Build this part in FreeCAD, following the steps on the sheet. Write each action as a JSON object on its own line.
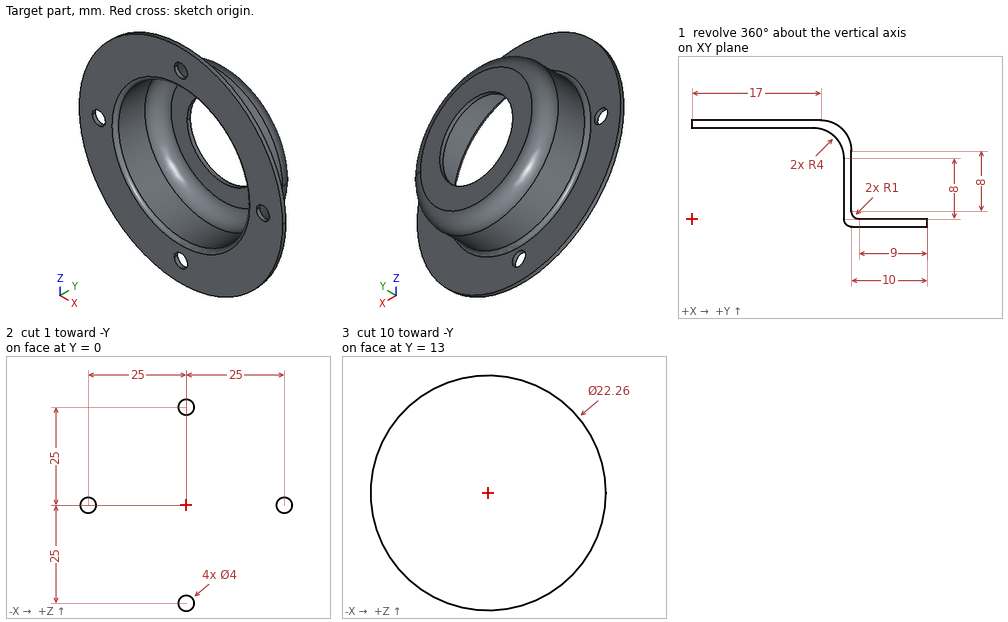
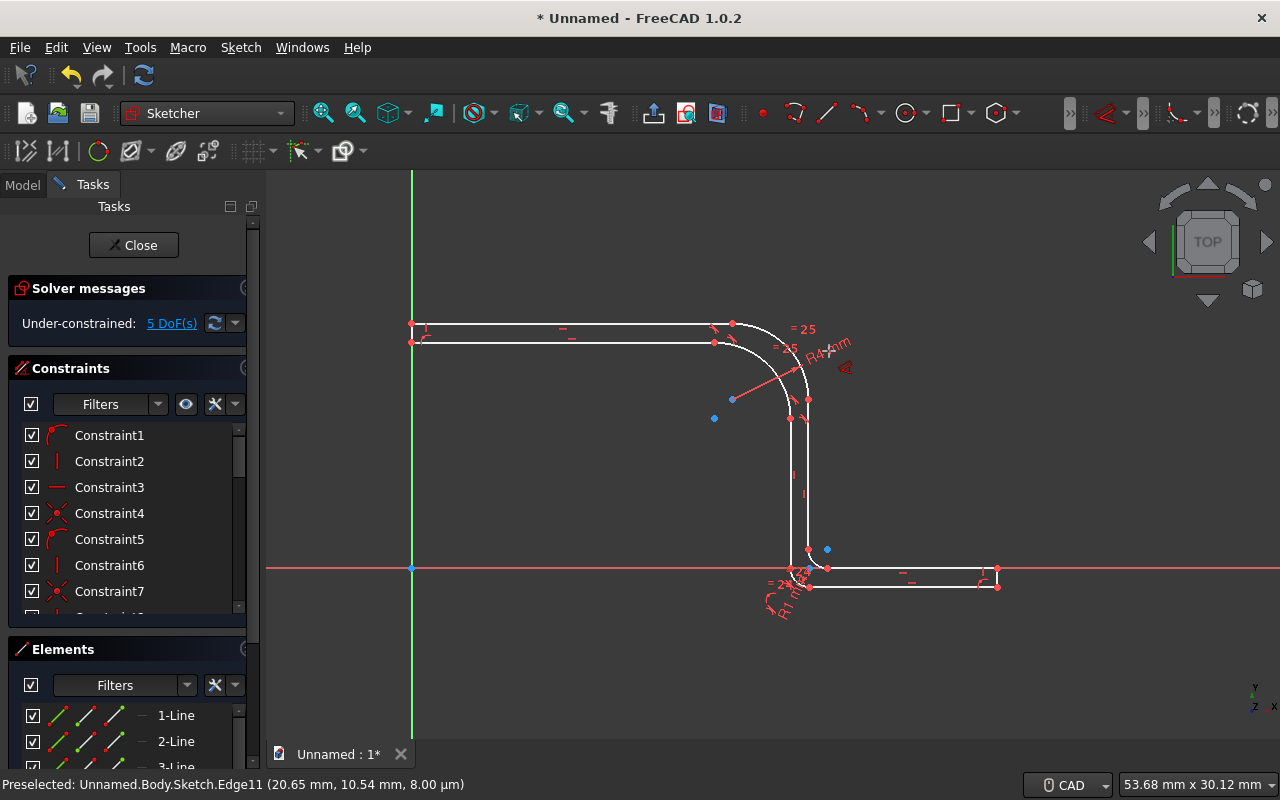
{"action": "left_click", "coordinate": [791, 463]}
{"action": "left_click", "coordinate": [825, 493]}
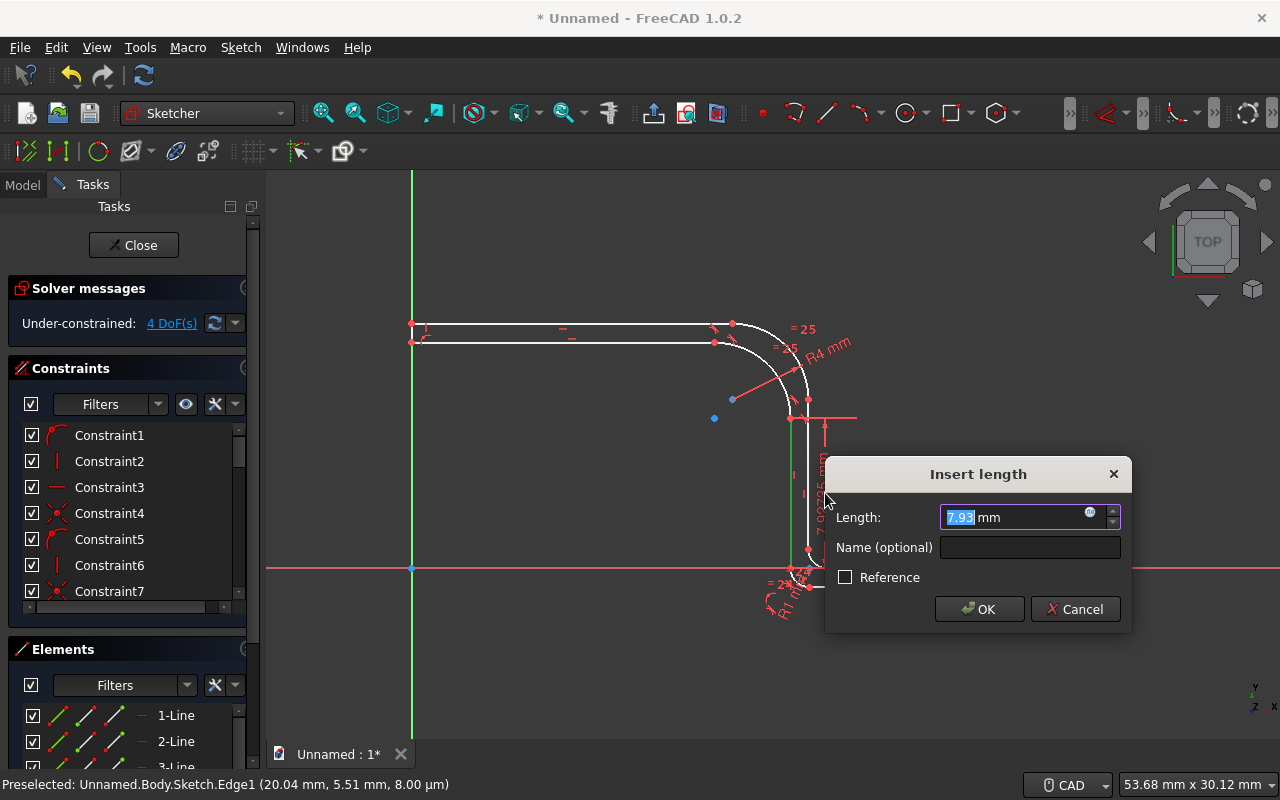
{"action": "type", "text": "8"}
{"action": "key", "text": "Return"}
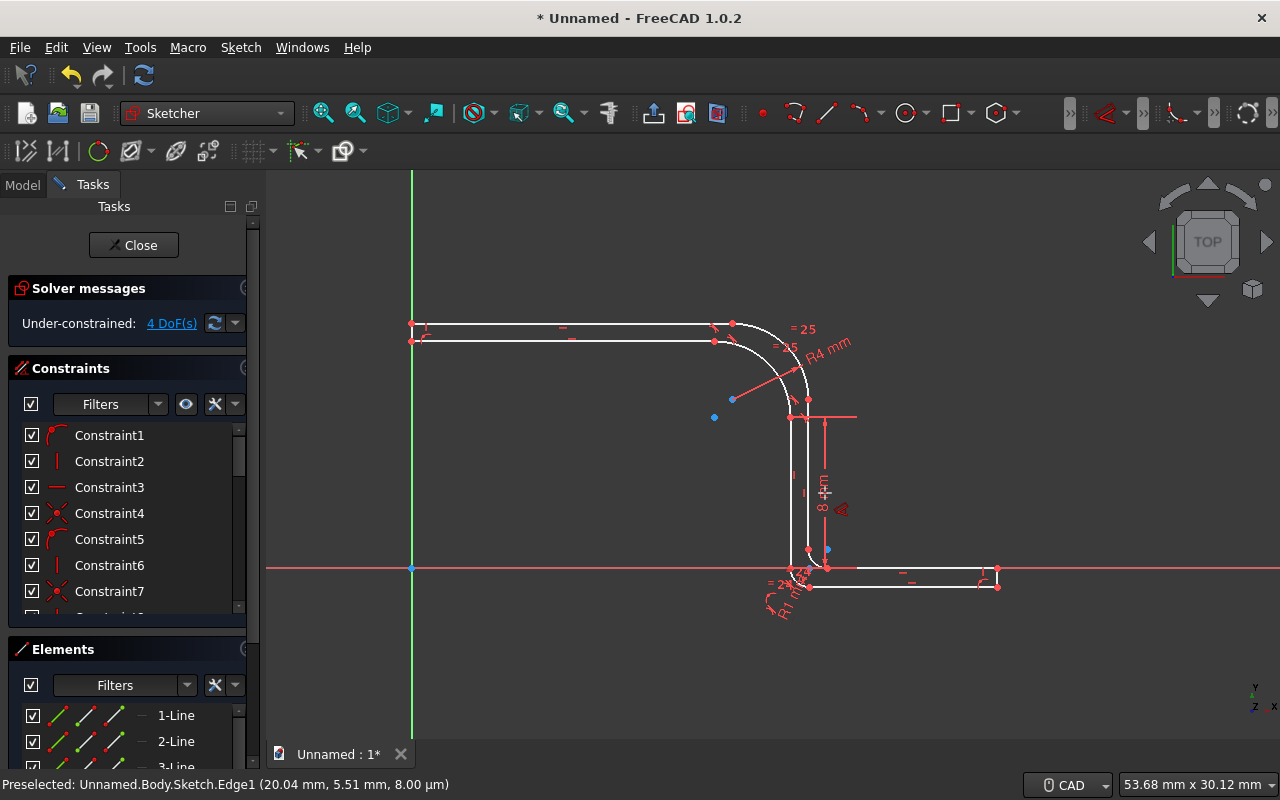
{"action": "left_click", "coordinate": [946, 568]}
{"action": "left_click", "coordinate": [912, 602]}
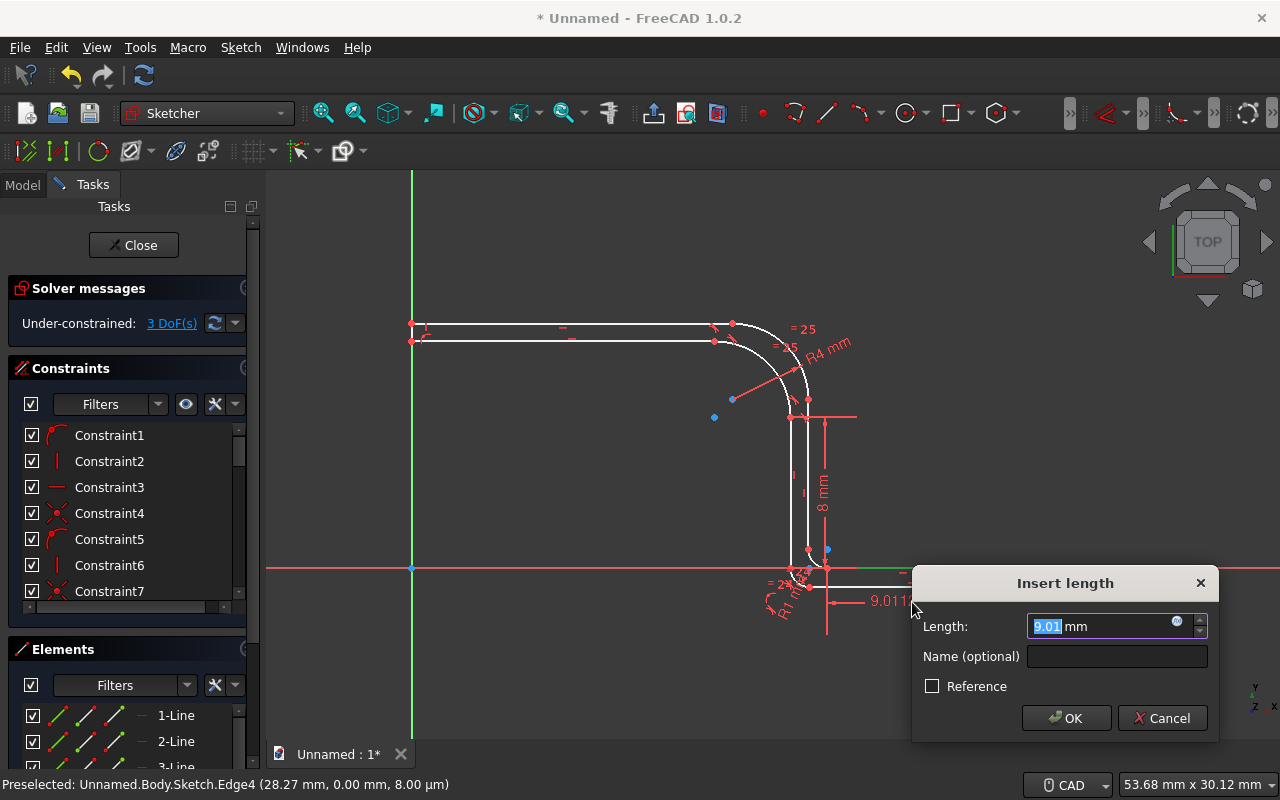
{"action": "type", "text": "9"}
{"action": "key", "text": "Return"}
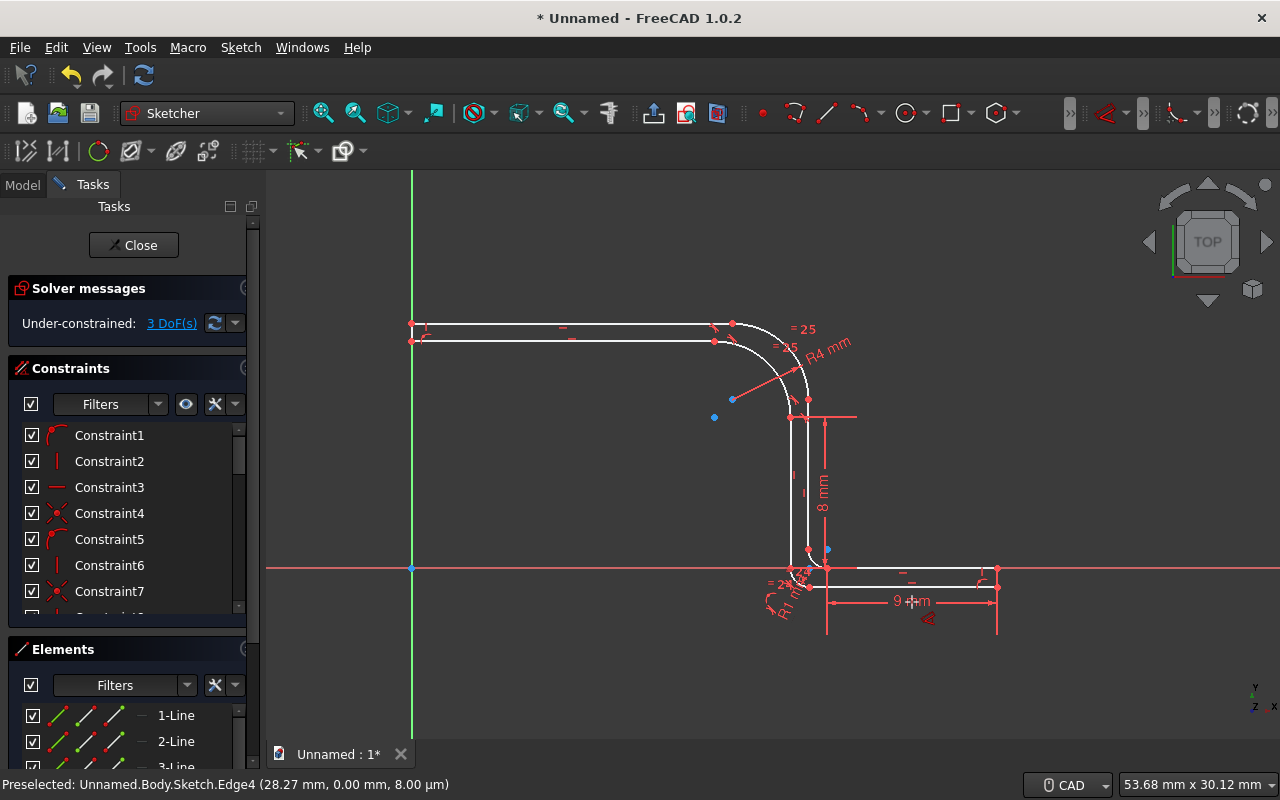
{"action": "left_click", "coordinate": [808, 504]}
{"action": "left_click", "coordinate": [842, 440]}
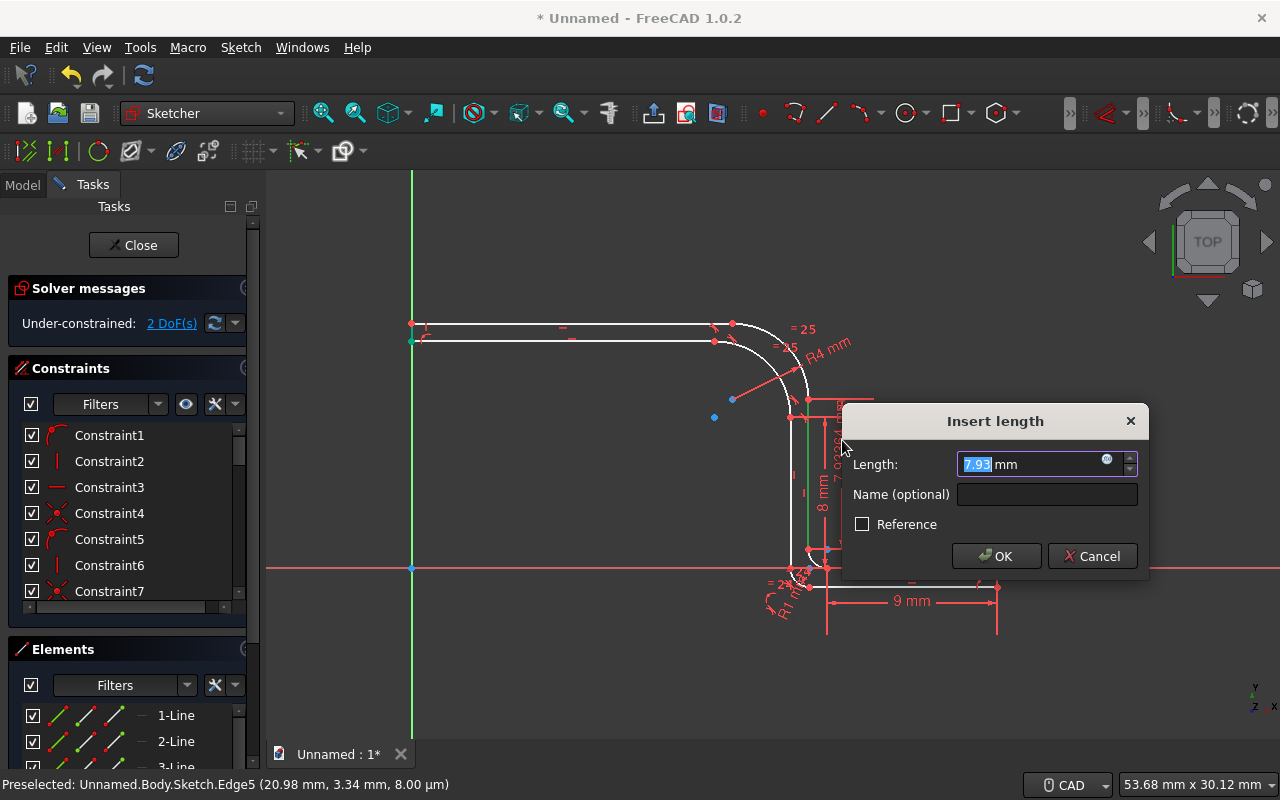
{"action": "type", "text": "8"}
{"action": "key", "text": "Return"}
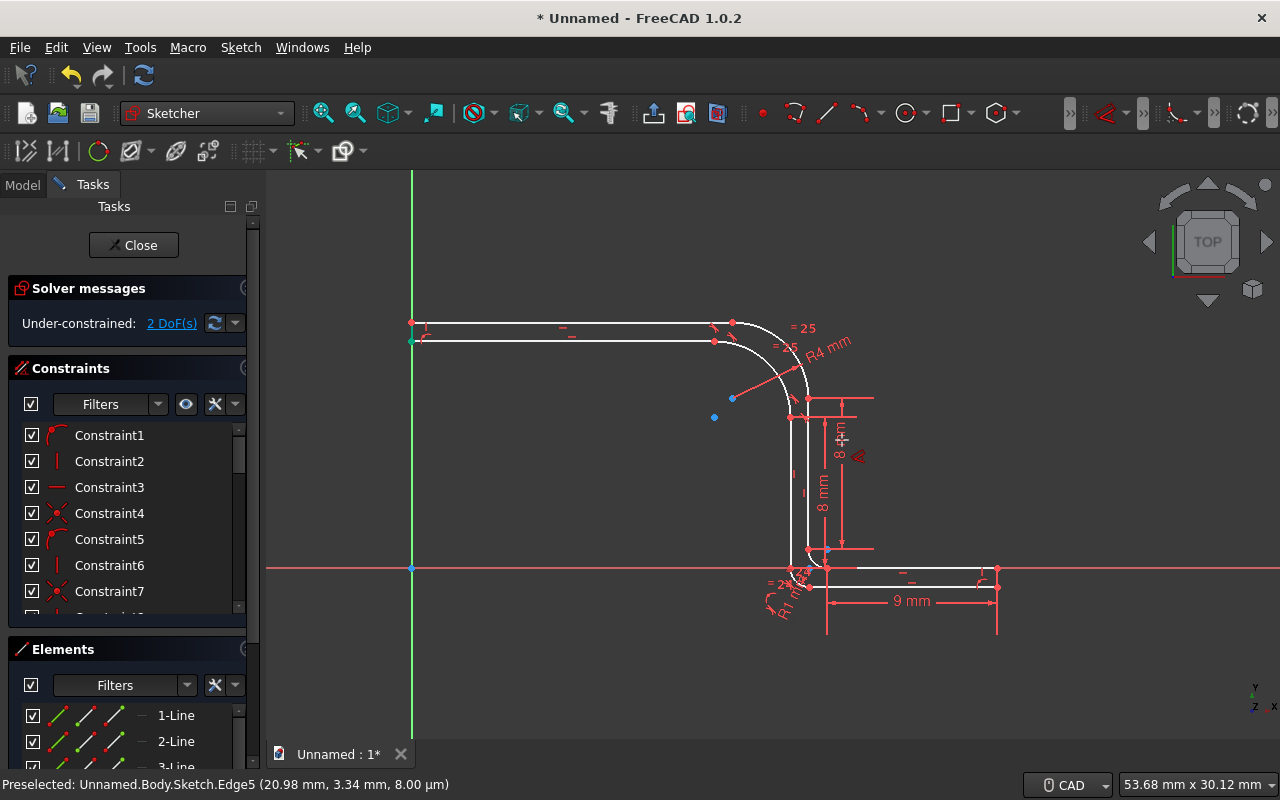
{"action": "left_click", "coordinate": [866, 587]}
{"action": "left_click", "coordinate": [838, 621]}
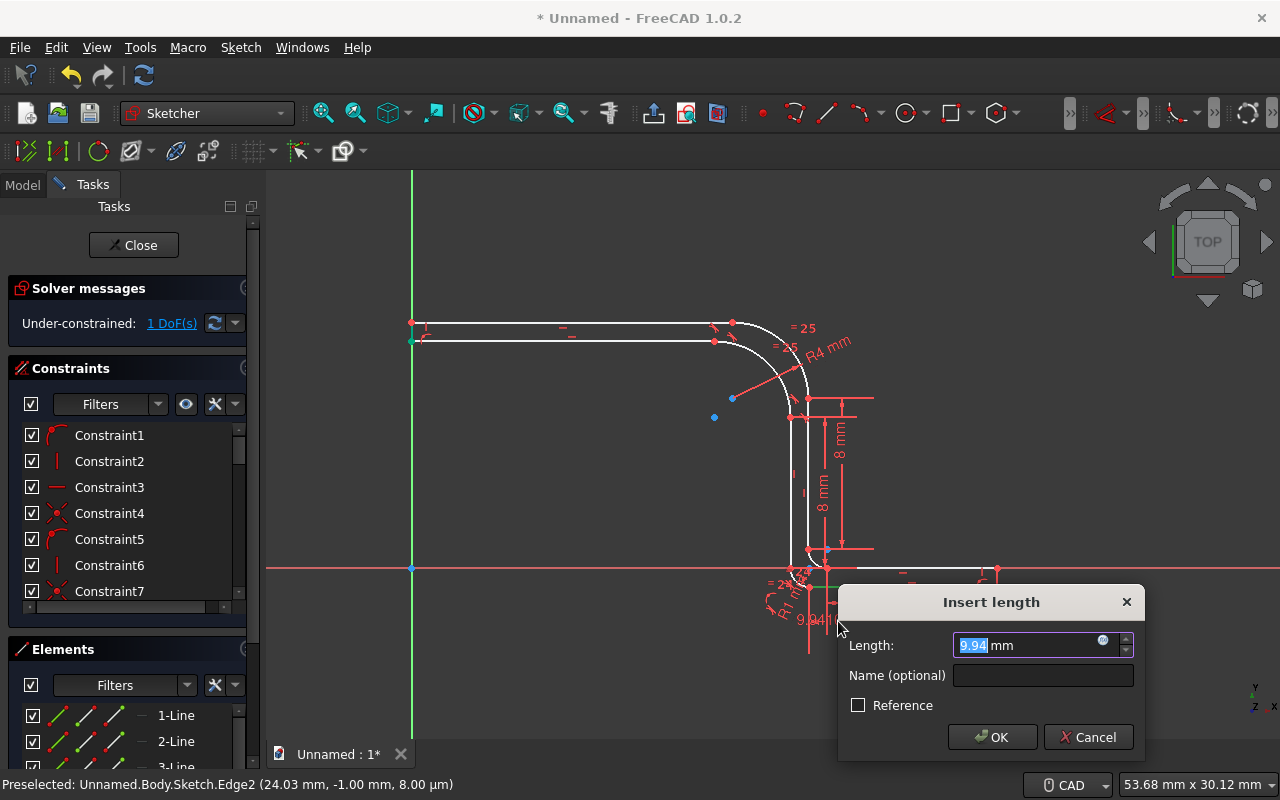
{"action": "type", "text": "10"}
{"action": "key", "text": "Return"}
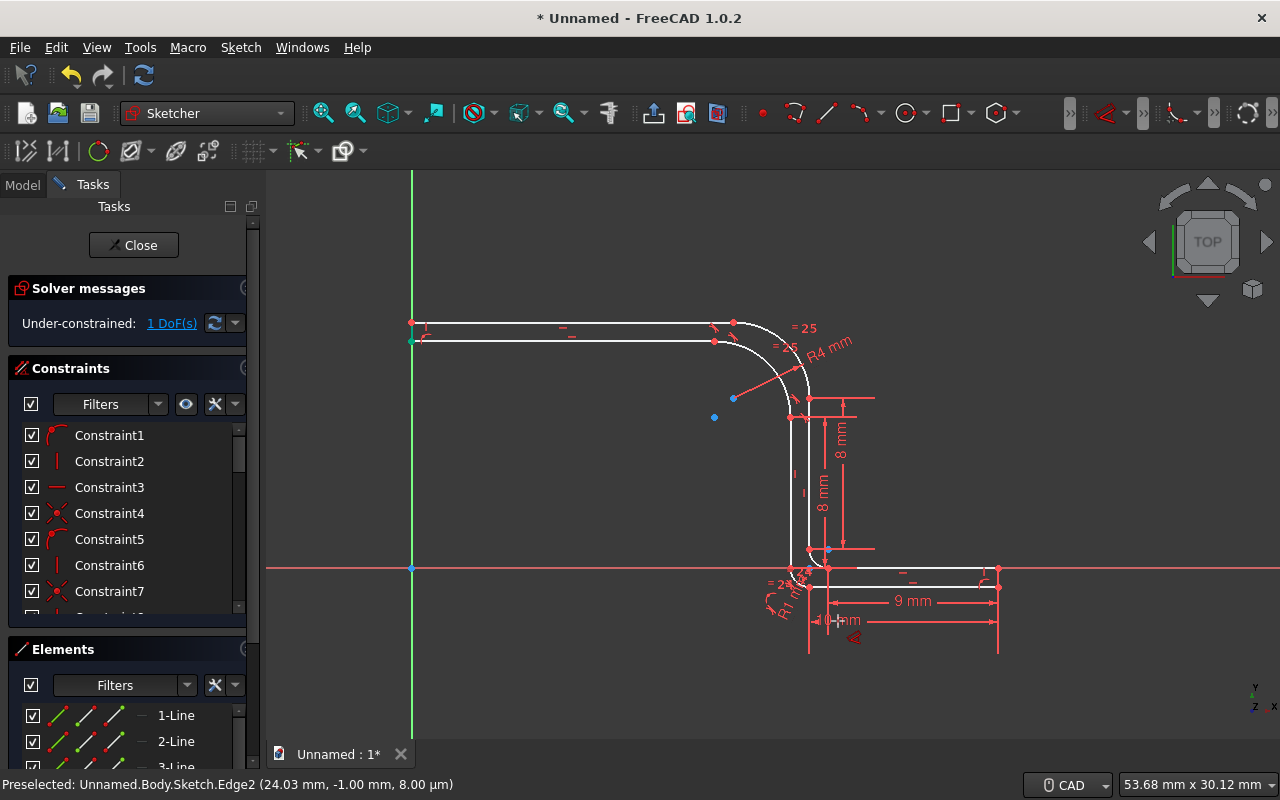
{"action": "left_click", "coordinate": [637, 323]}
{"action": "left_click", "coordinate": [573, 289]}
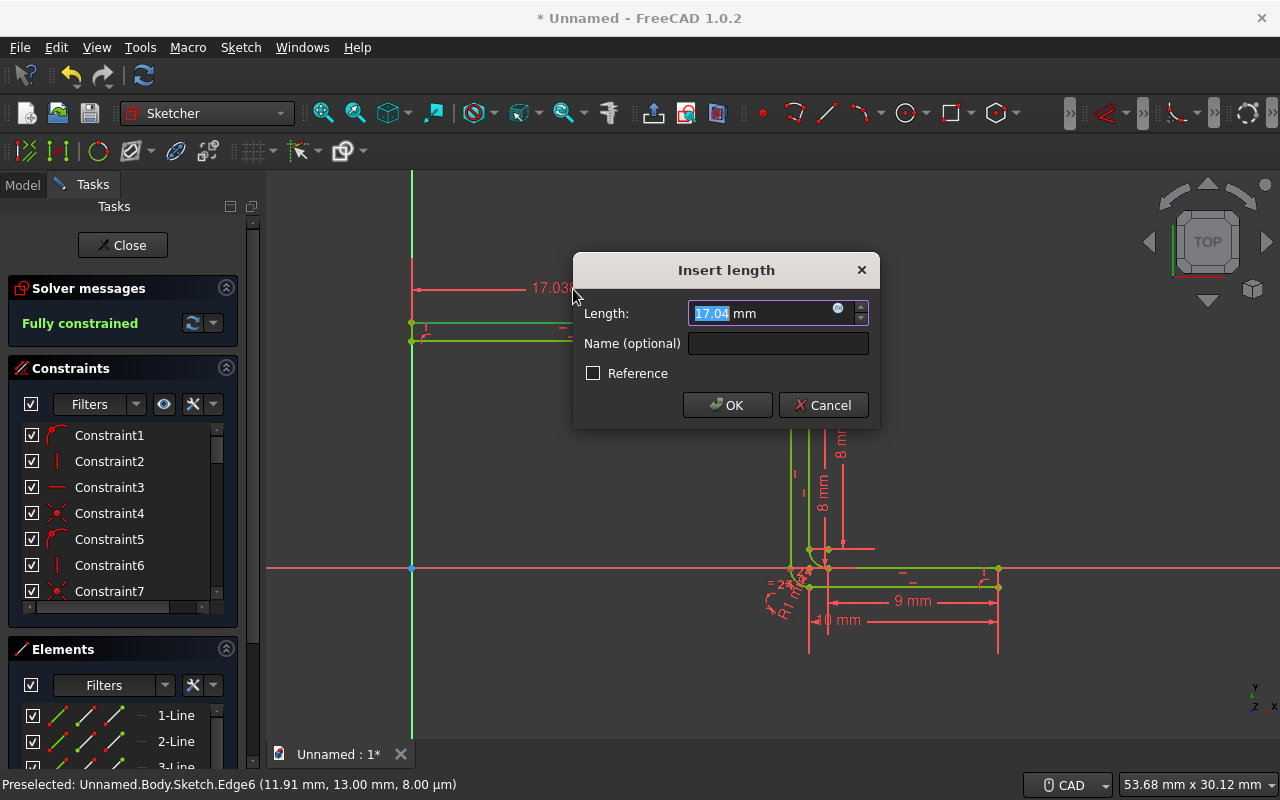
{"action": "type", "text": "17"}
{"action": "key", "text": "Return"}
{"action": "key", "text": "Escape"}